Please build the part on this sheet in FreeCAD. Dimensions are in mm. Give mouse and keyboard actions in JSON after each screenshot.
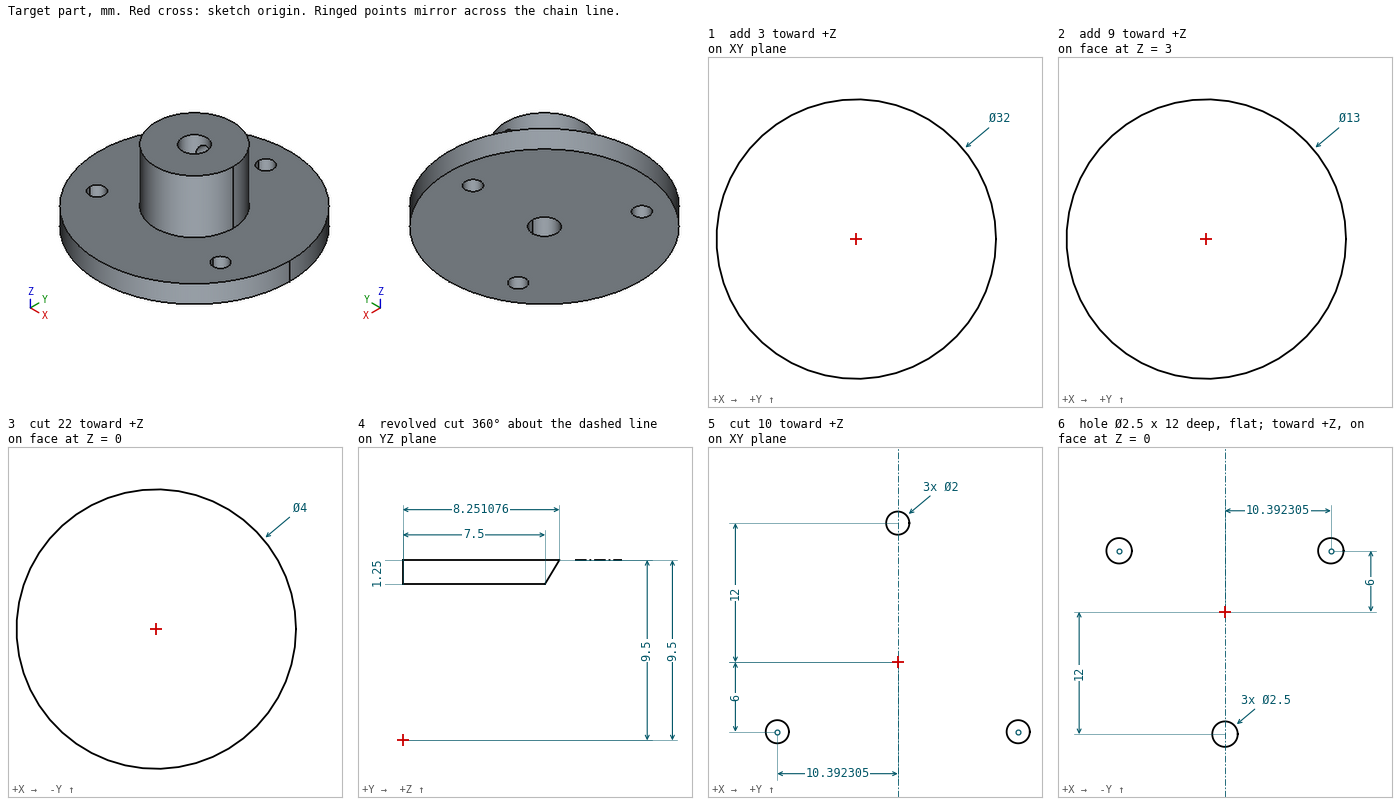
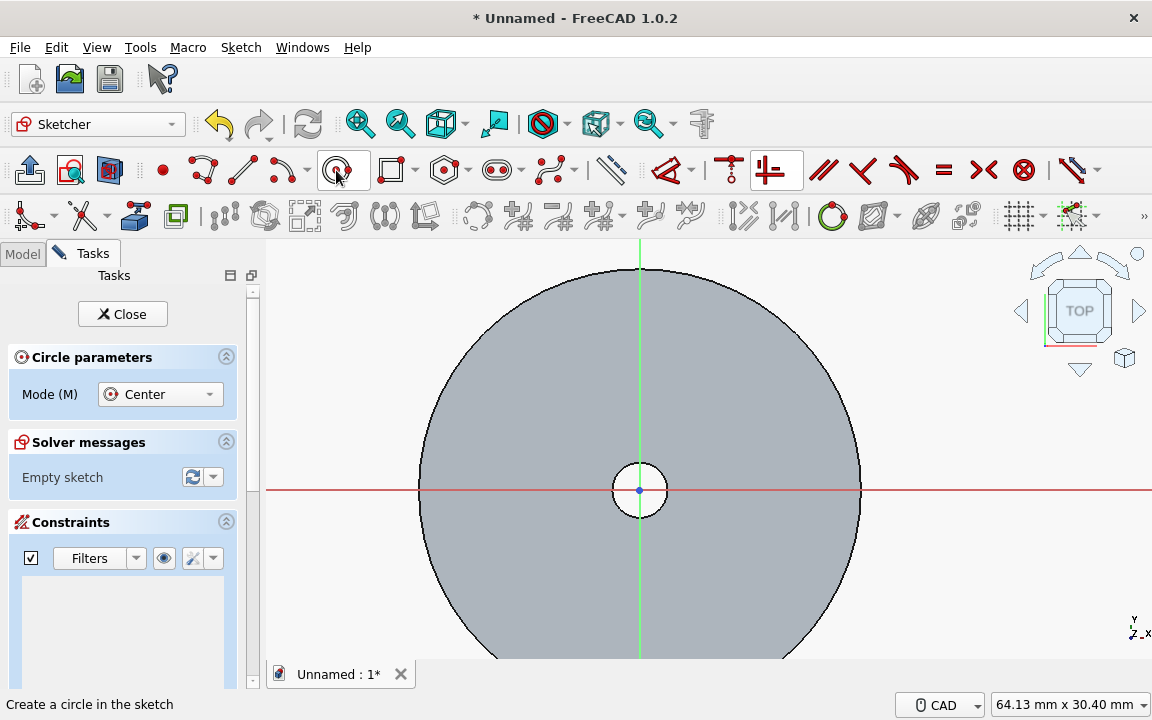
{"action": "scroll", "coordinate": [640, 324], "scroll_direction": "up", "scroll_amount": 3}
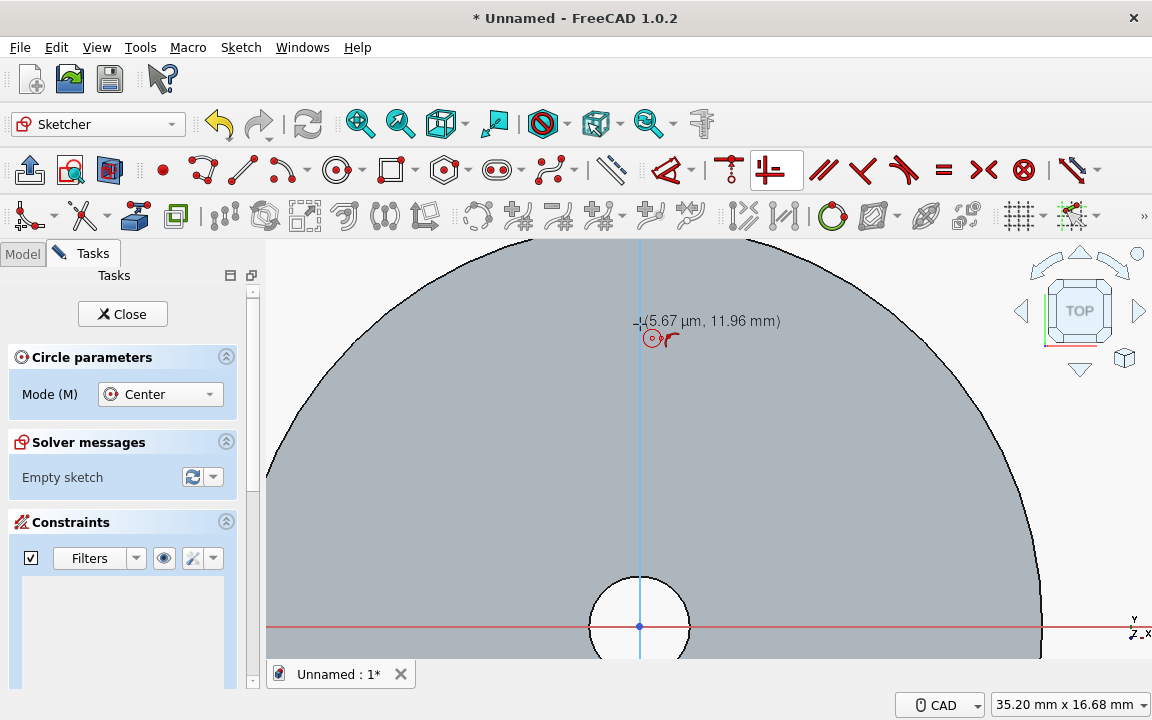
{"action": "left_click", "coordinate": [640, 325]}
{"action": "mouse_move", "coordinate": [657, 307]}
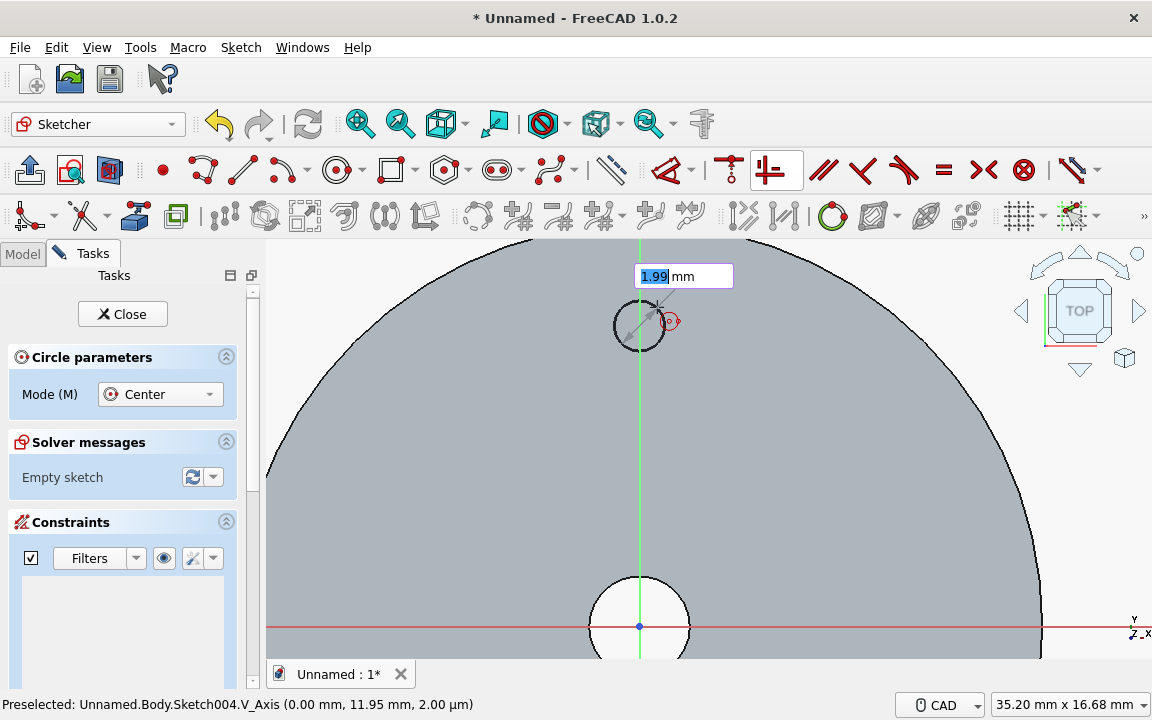
{"action": "type", "text": "2"}
{"action": "key", "text": "Return"}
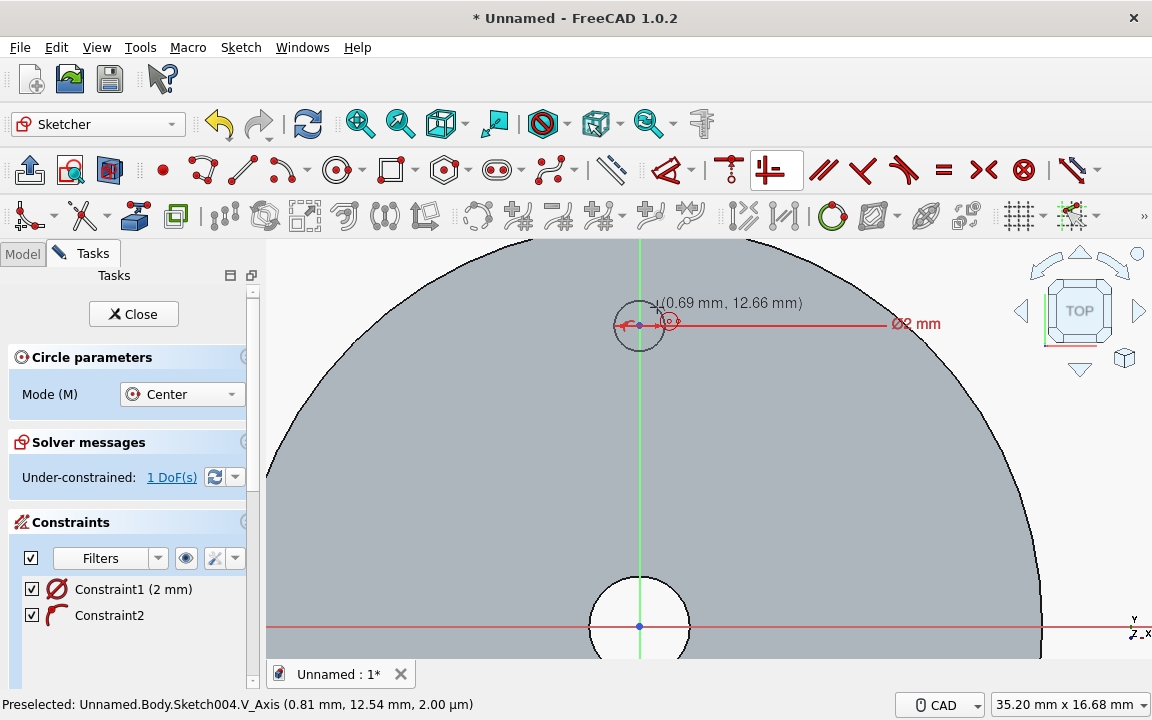
{"action": "scroll", "coordinate": [642, 325], "scroll_direction": "down", "scroll_amount": 3}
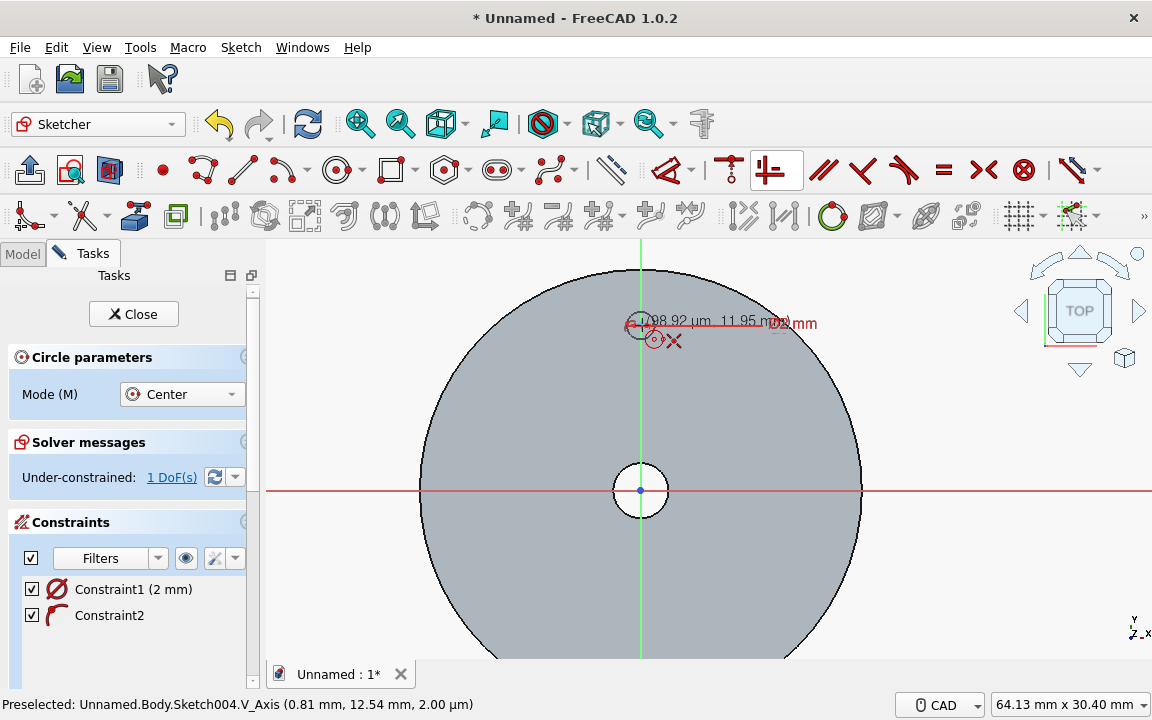
{"action": "scroll", "coordinate": [497, 574], "scroll_direction": "up", "scroll_amount": 3}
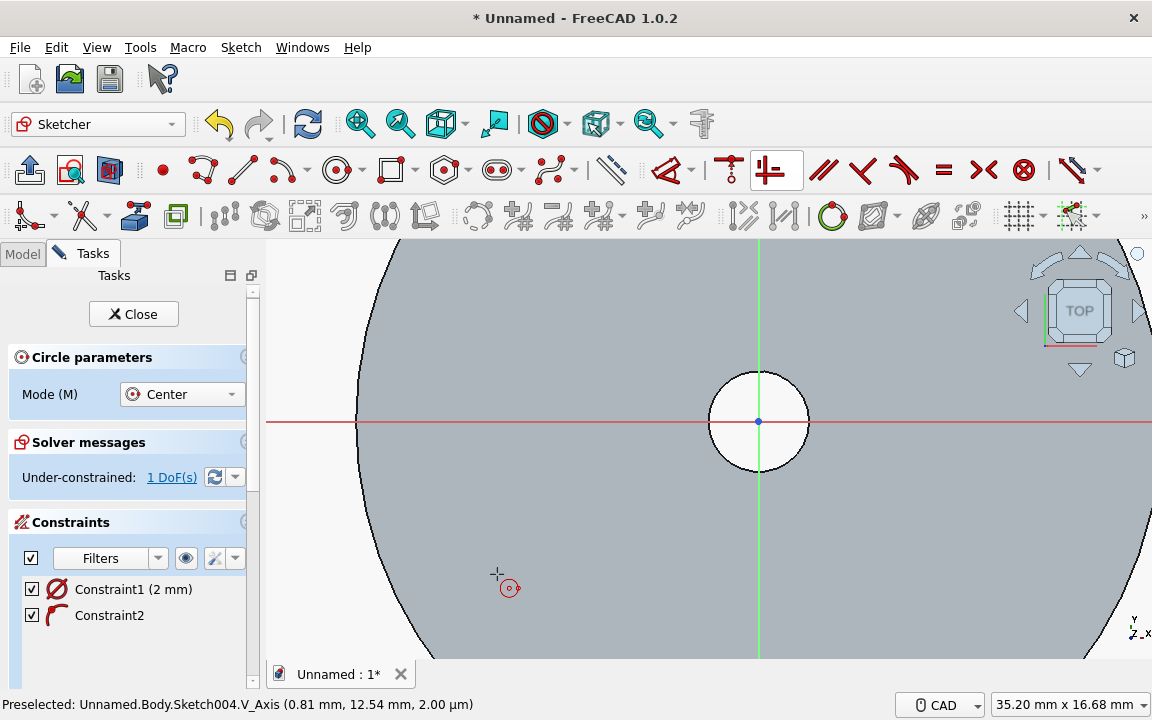
{"action": "left_click", "coordinate": [497, 573]}
{"action": "mouse_move", "coordinate": [515, 555]}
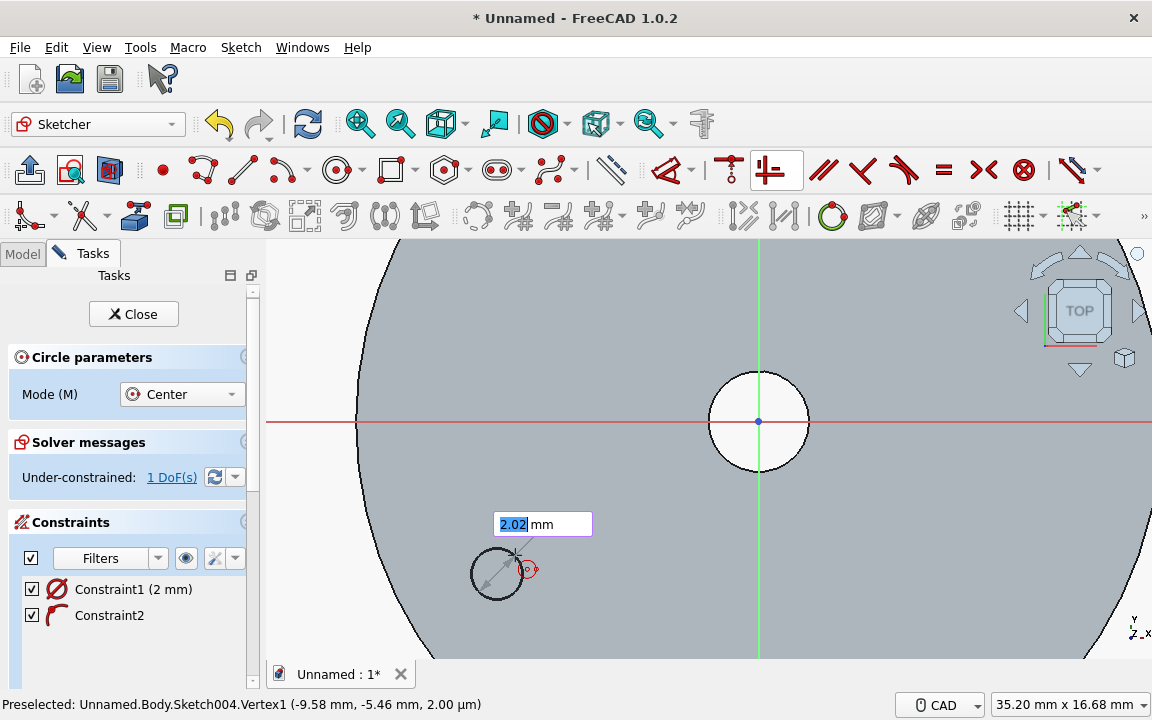
{"action": "type", "text": "2"}
{"action": "key", "text": "Return"}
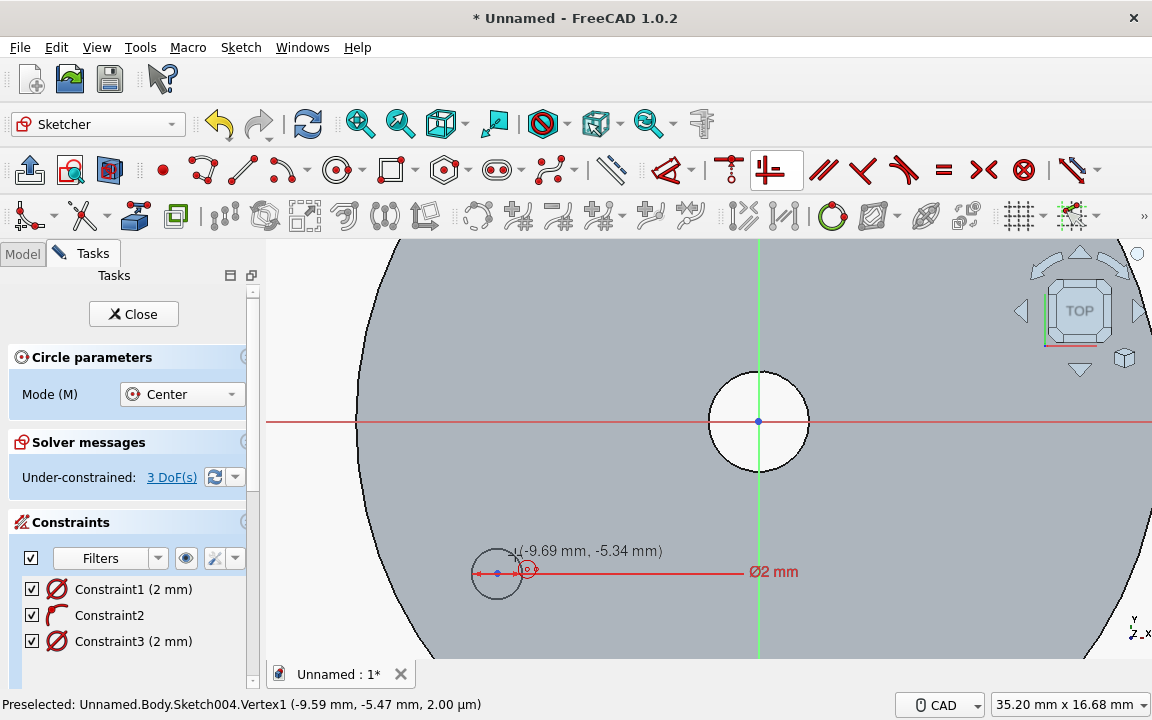
{"action": "scroll", "coordinate": [497, 574], "scroll_direction": "down", "scroll_amount": 3}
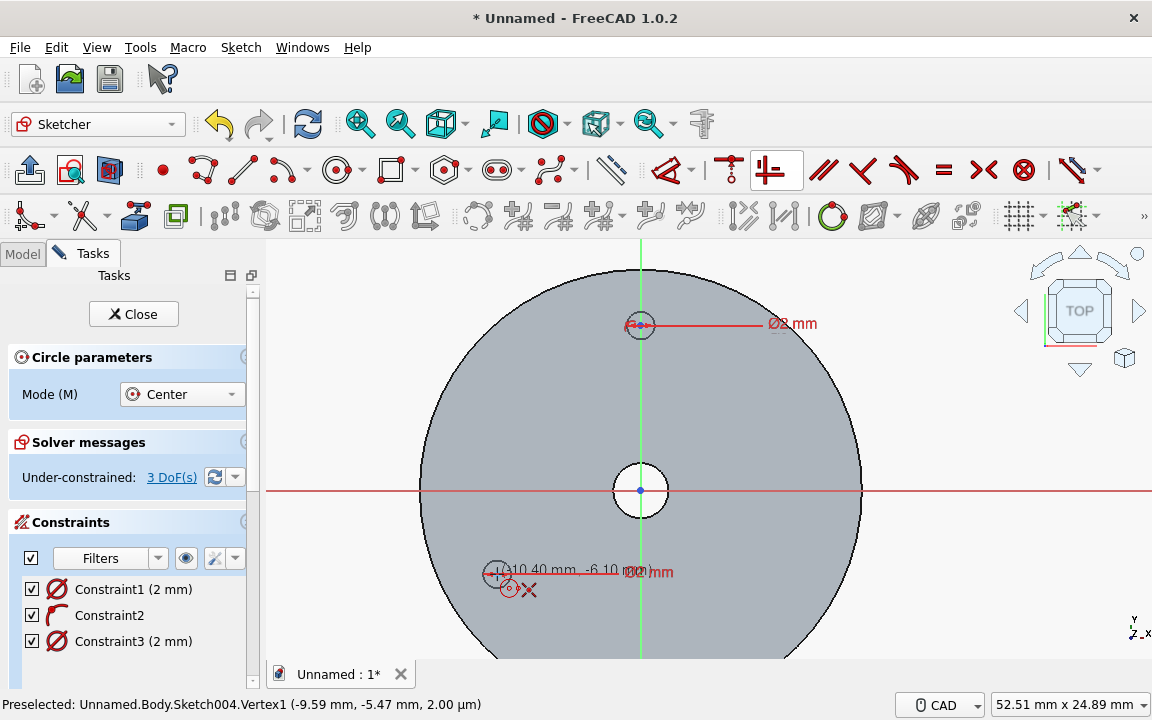
{"action": "scroll", "coordinate": [784, 574], "scroll_direction": "up", "scroll_amount": 3}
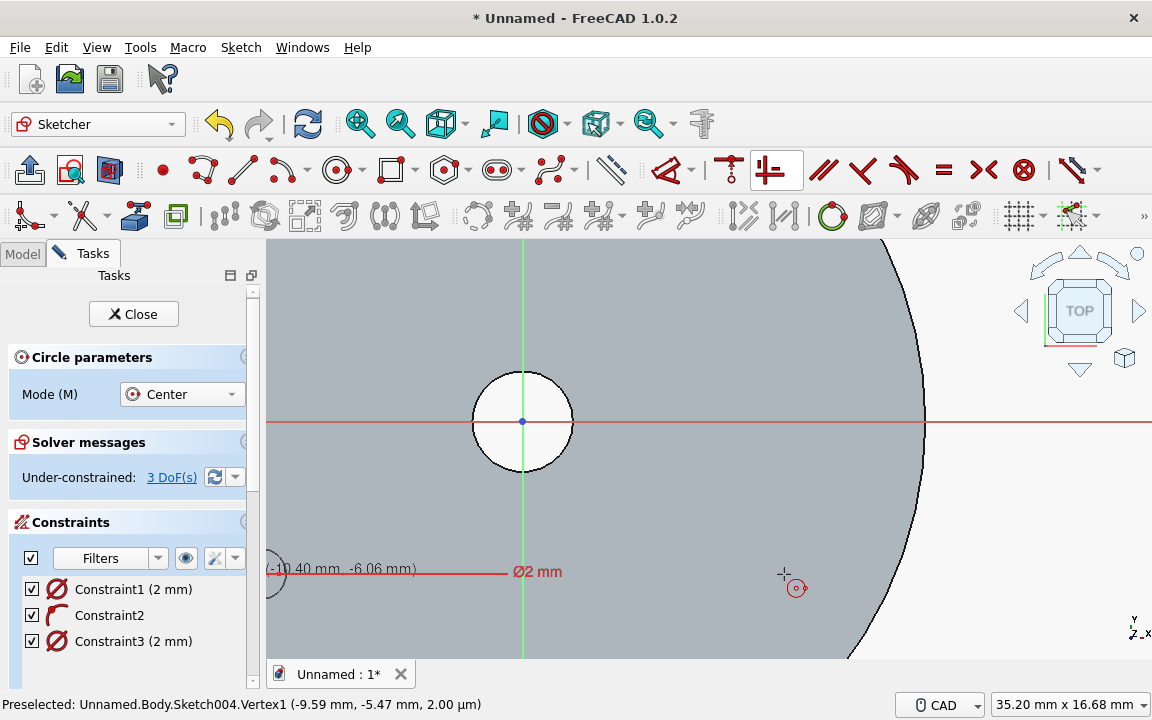
{"action": "left_click", "coordinate": [784, 573]}
{"action": "mouse_move", "coordinate": [802, 555]}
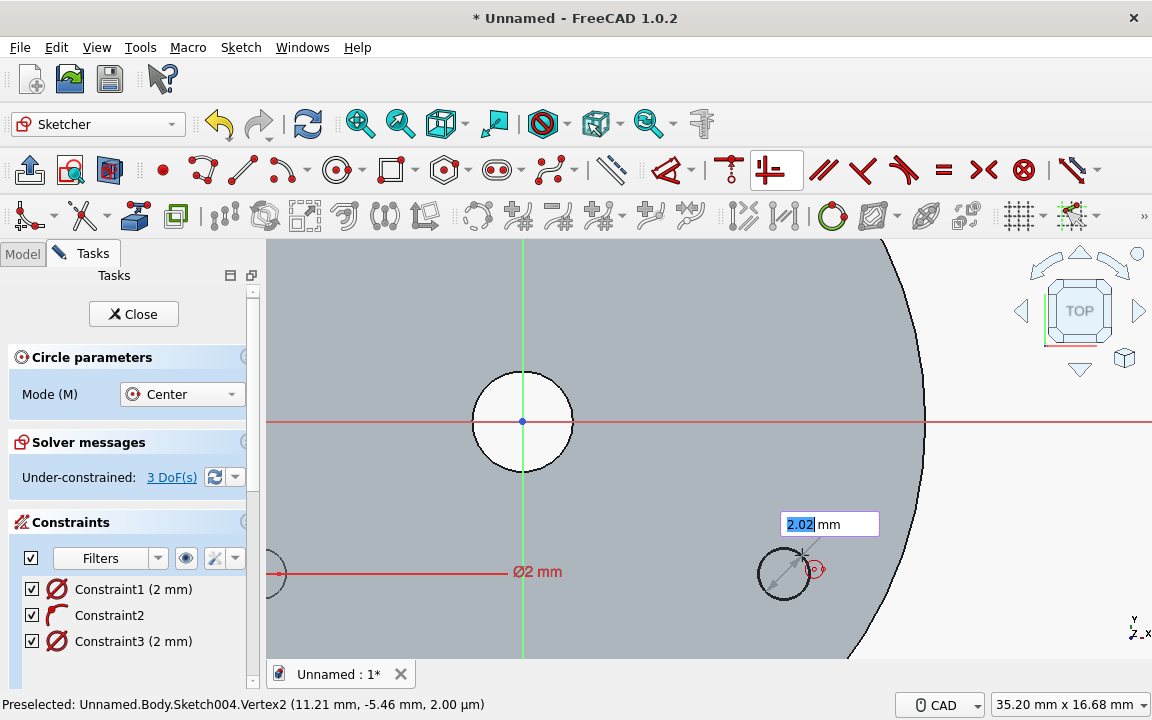
{"action": "type", "text": "2"}
{"action": "key", "text": "Return"}
{"action": "key", "text": "Escape"}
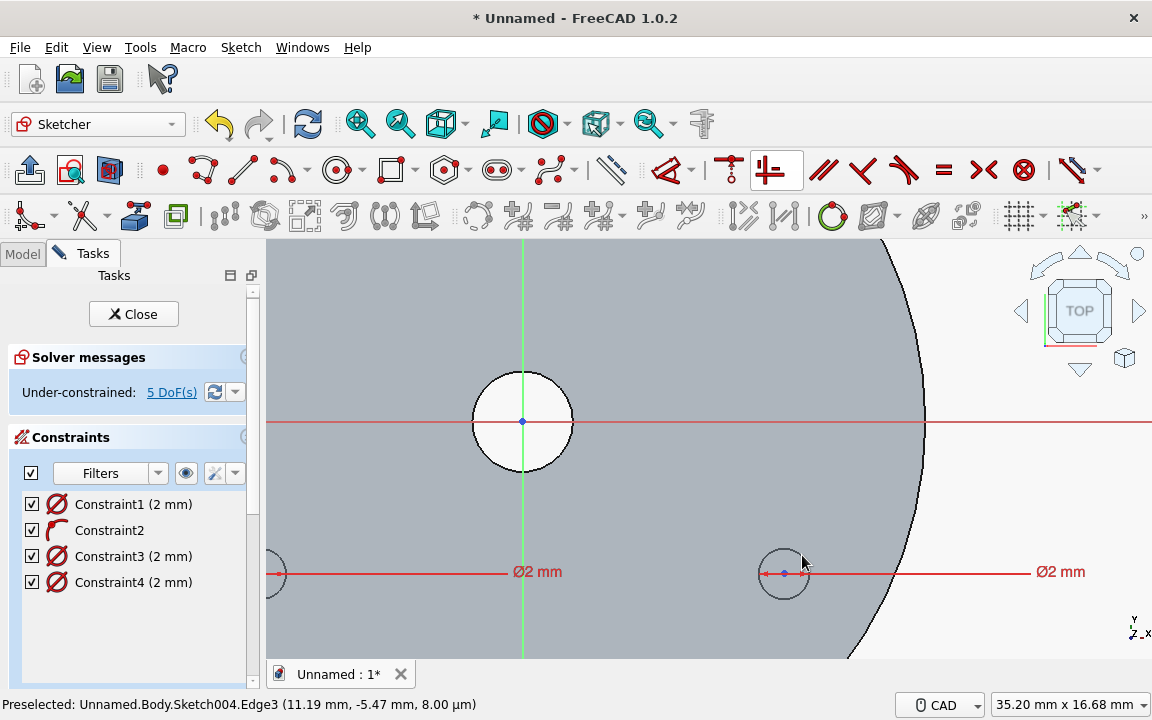
{"action": "scroll", "coordinate": [784, 574], "scroll_direction": "down", "scroll_amount": 3}